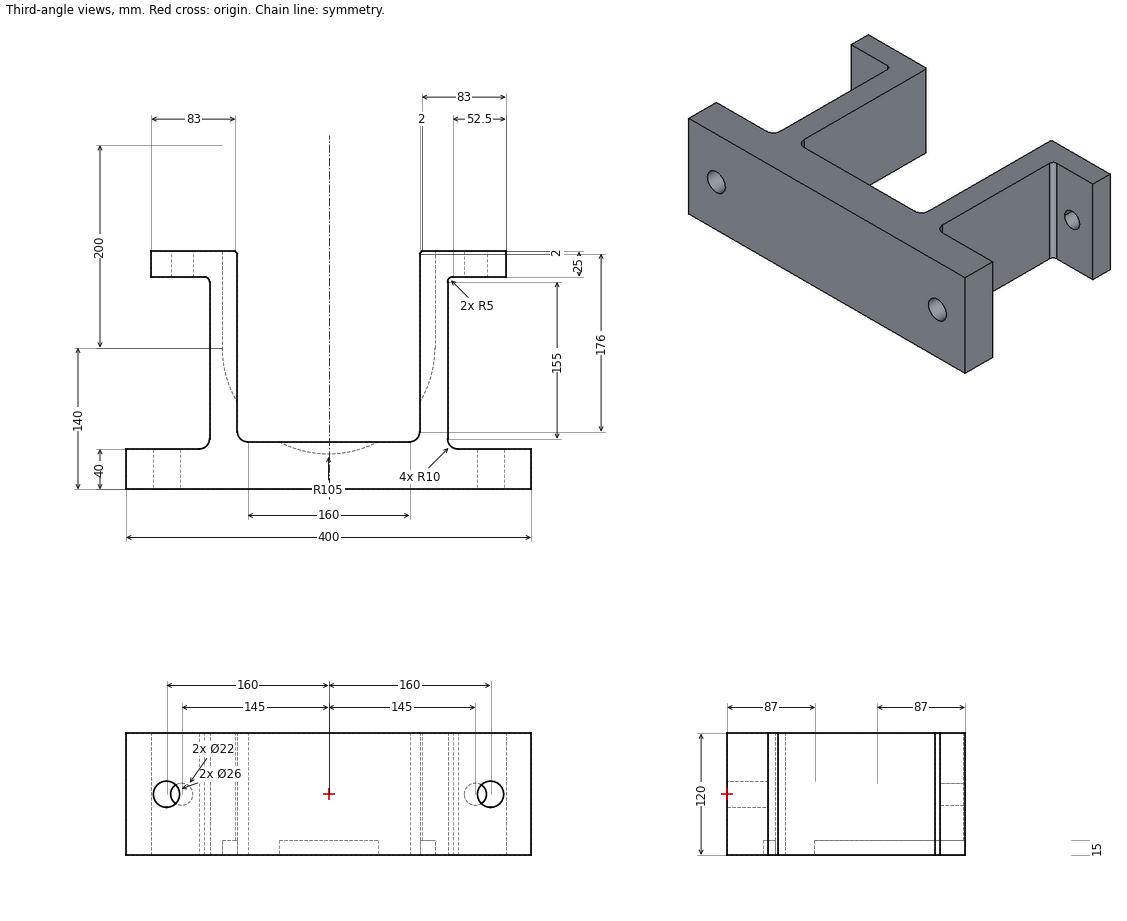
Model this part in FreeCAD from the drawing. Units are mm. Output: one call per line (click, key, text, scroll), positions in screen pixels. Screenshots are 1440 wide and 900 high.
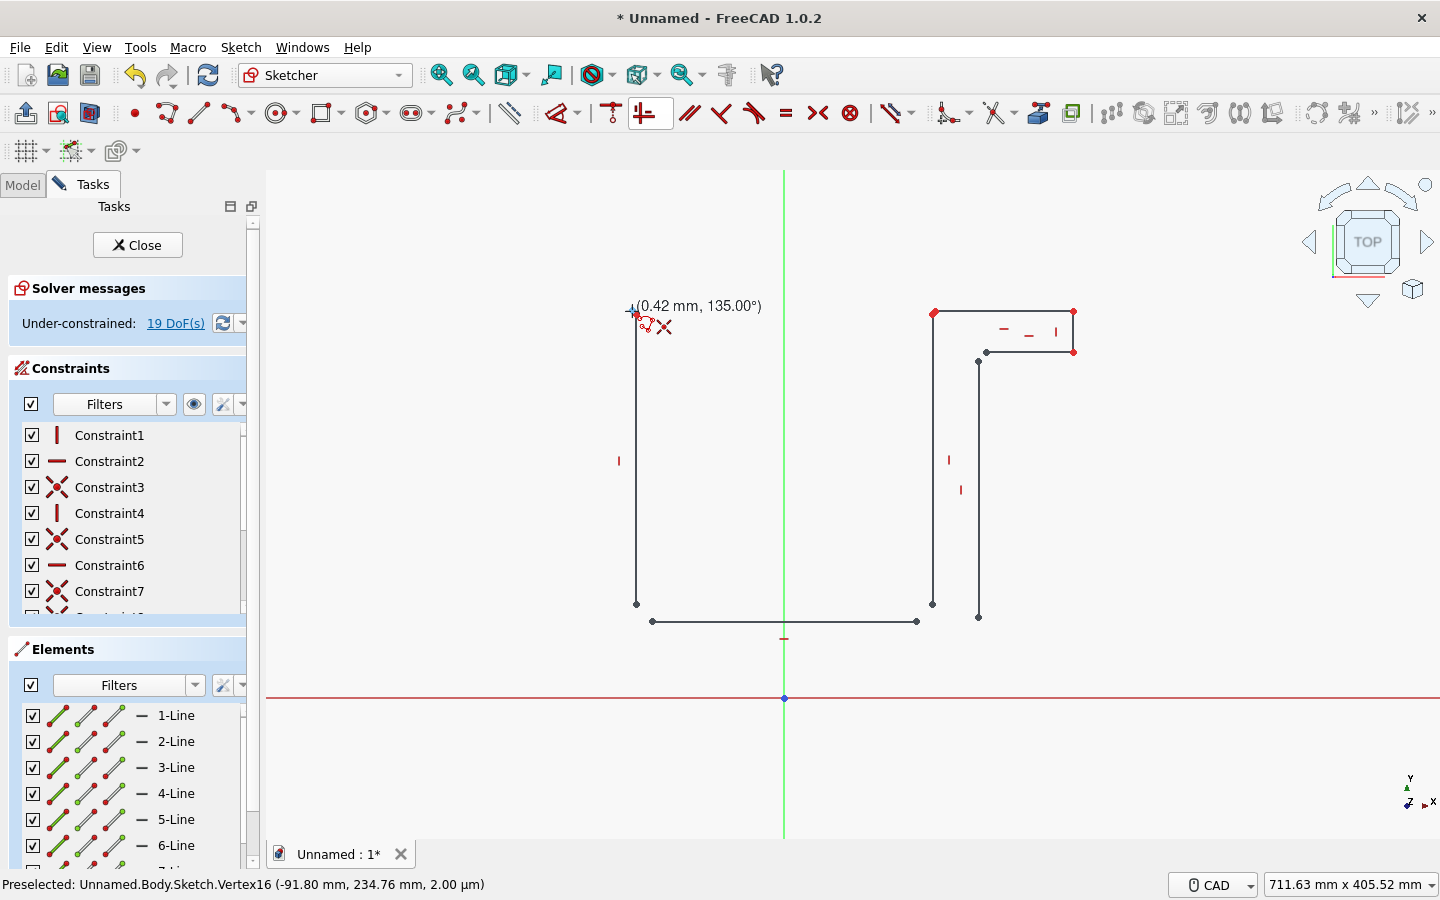
click(496, 311)
click(496, 352)
click(582, 352)
right_click(582, 352)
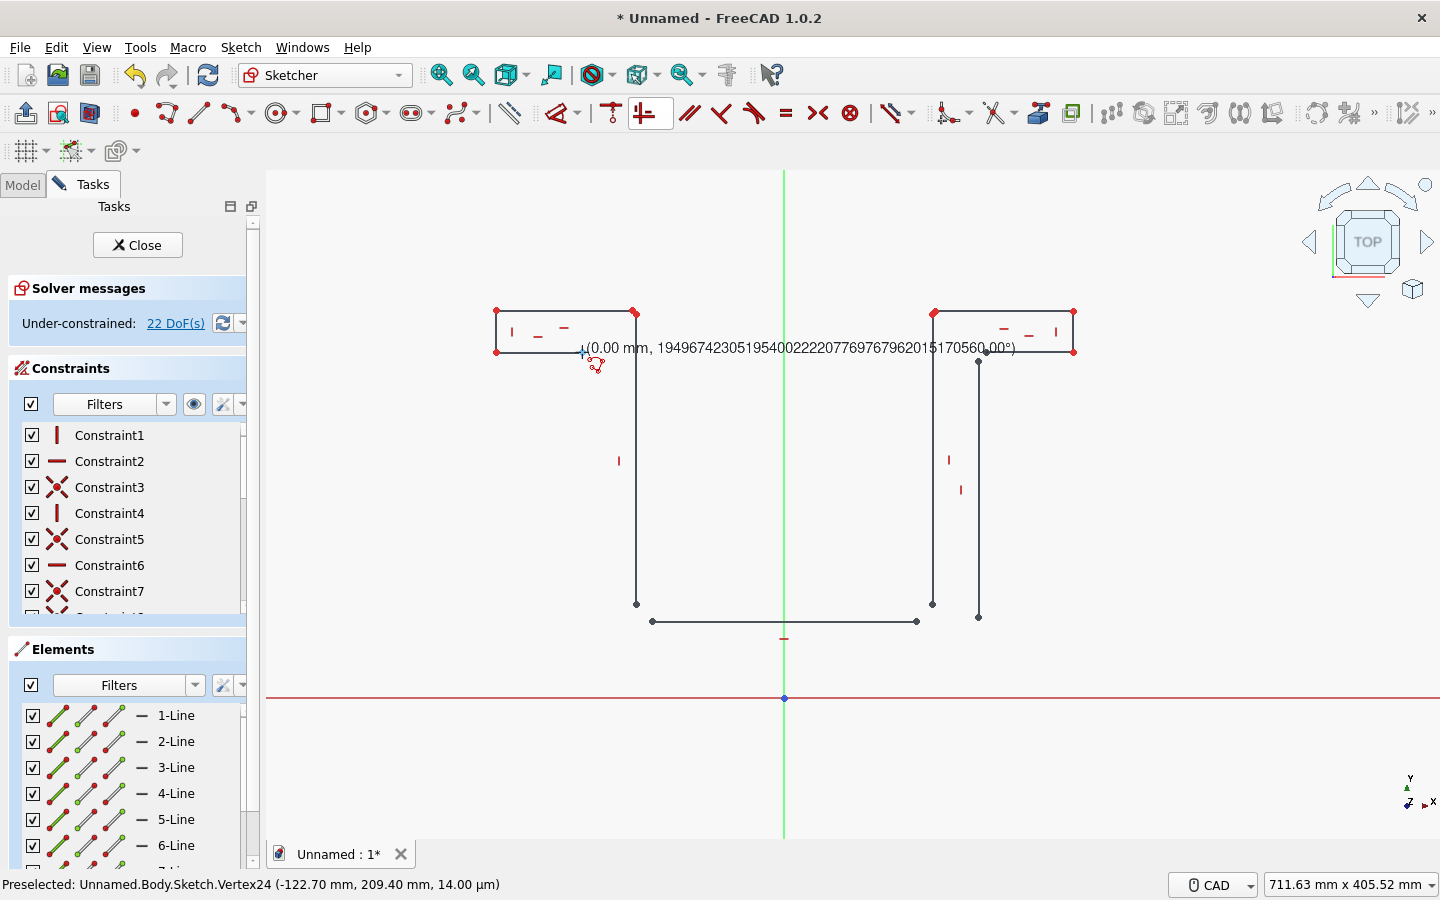
click(200, 114)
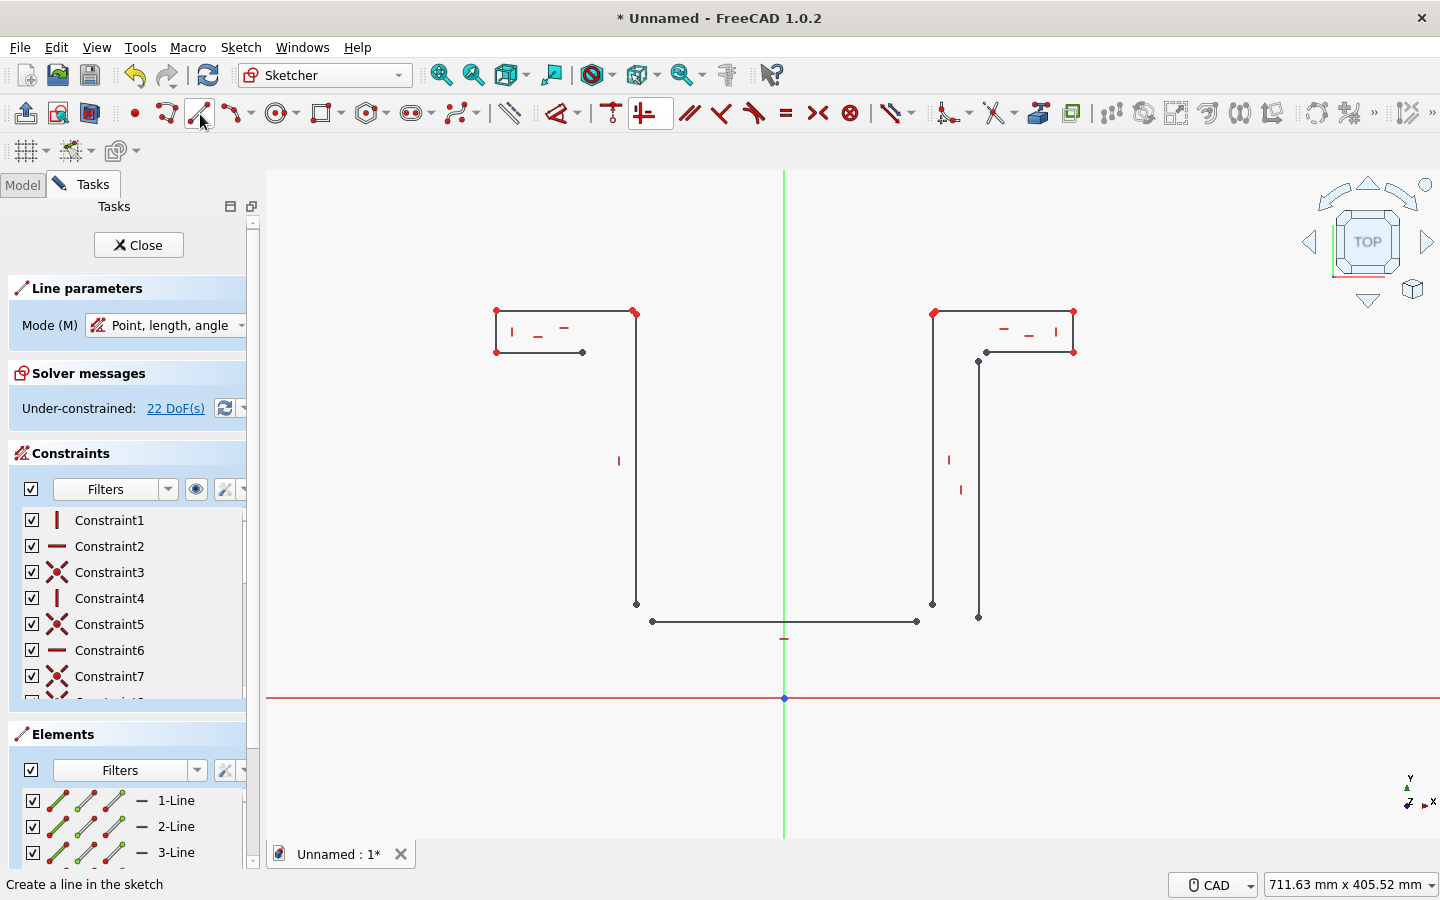
scroll(591, 360, up, 2)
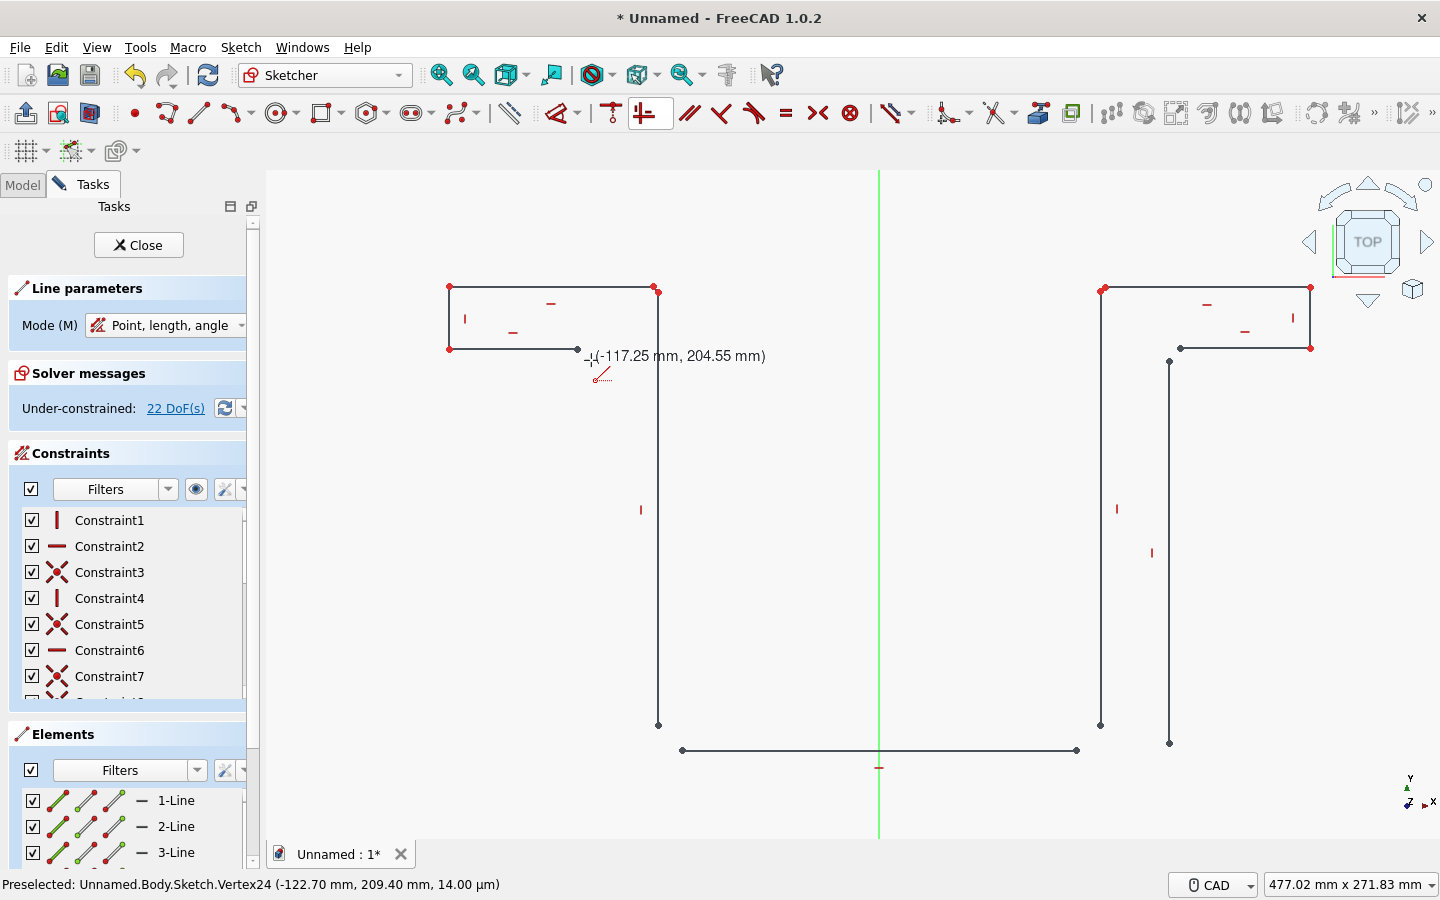
click(590, 360)
click(590, 742)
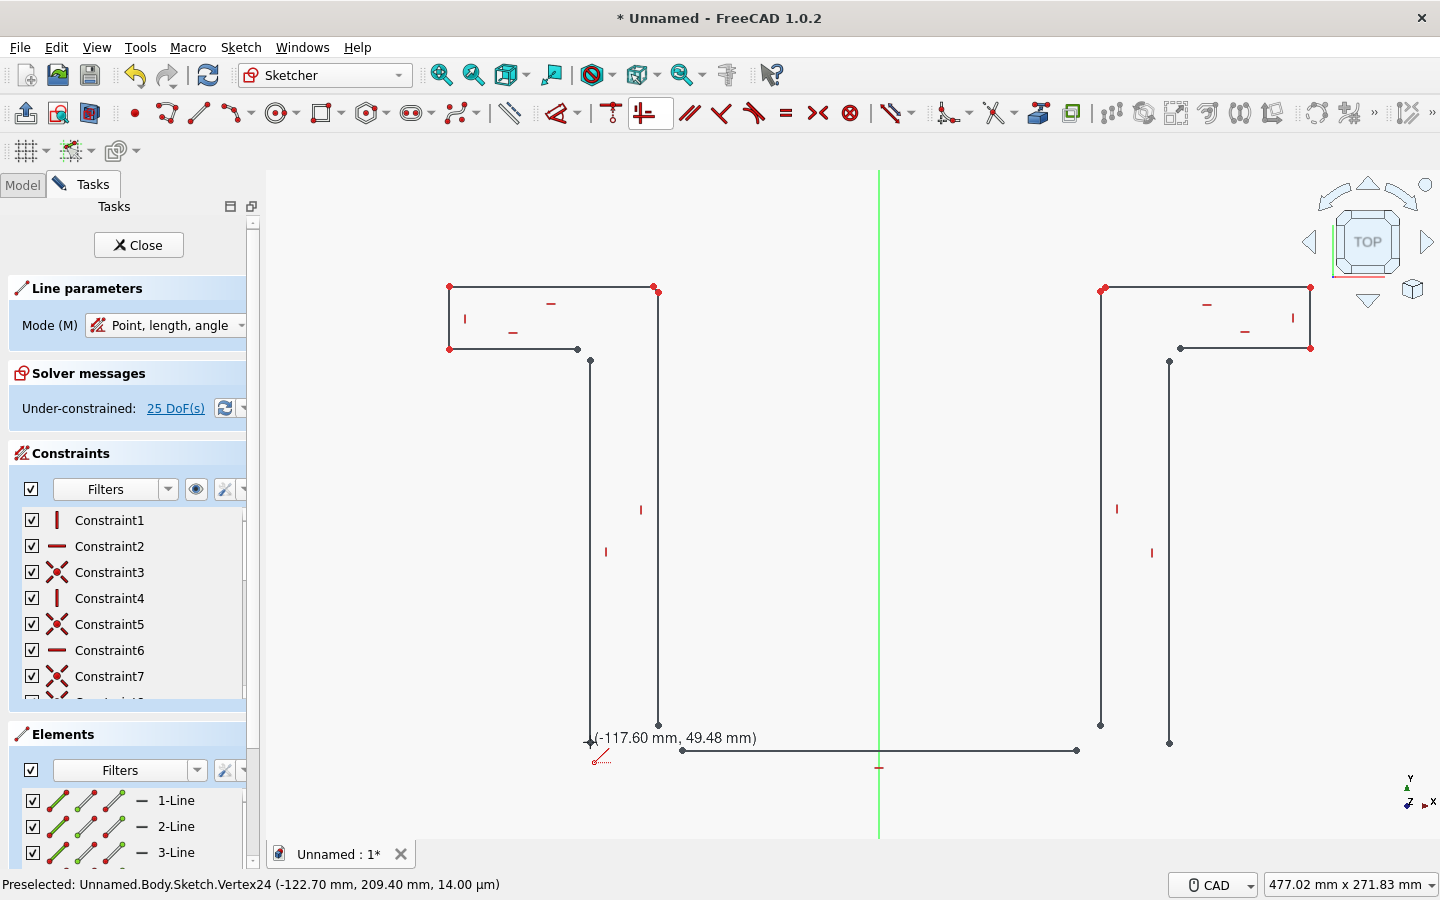
click(168, 114)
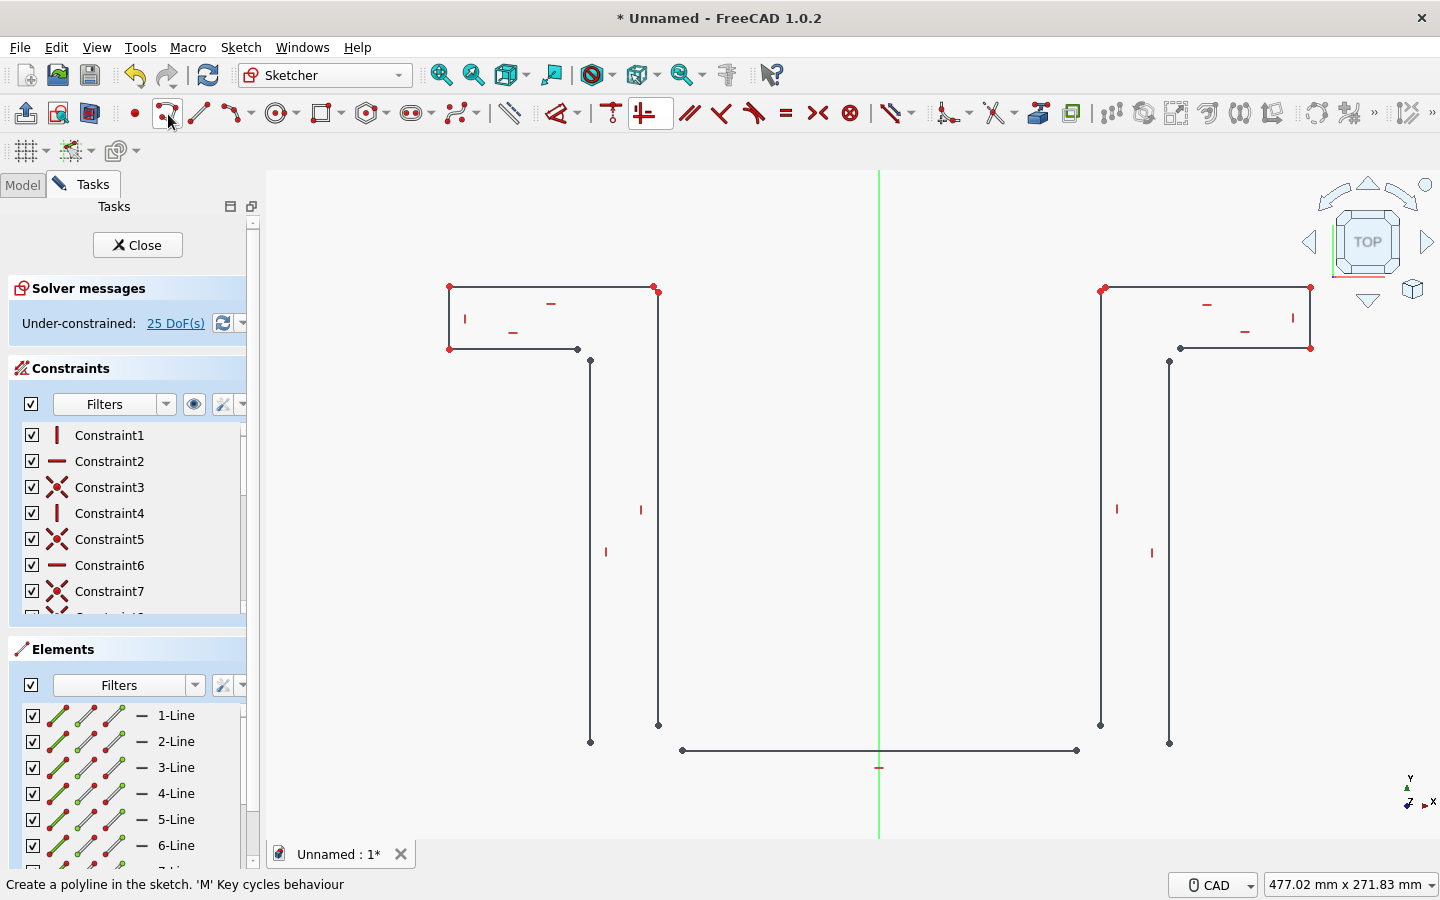
click(566, 766)
click(387, 766)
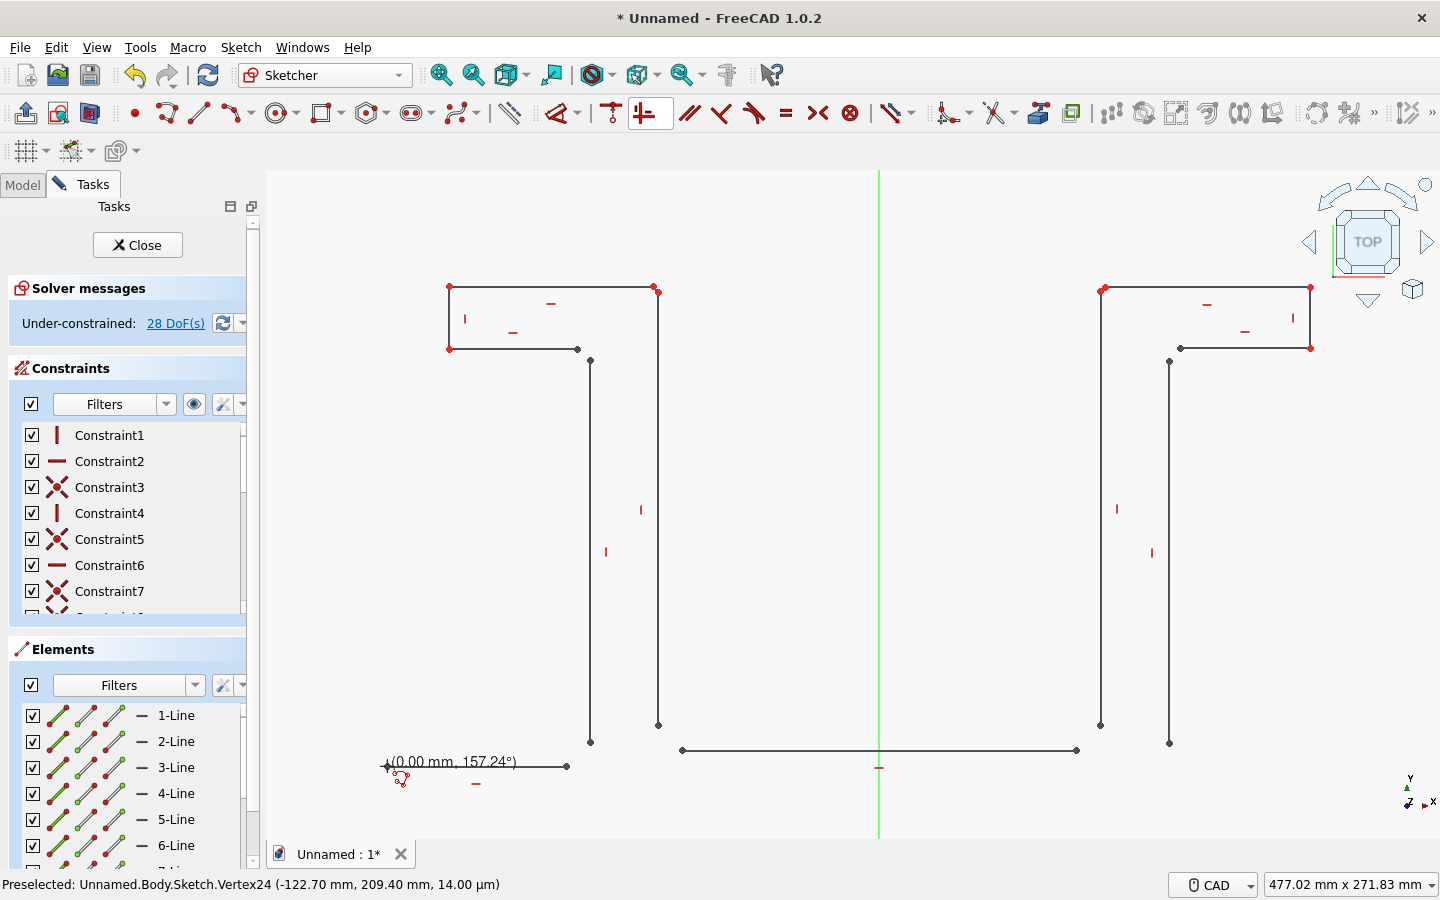
scroll(592, 360, down, 2)